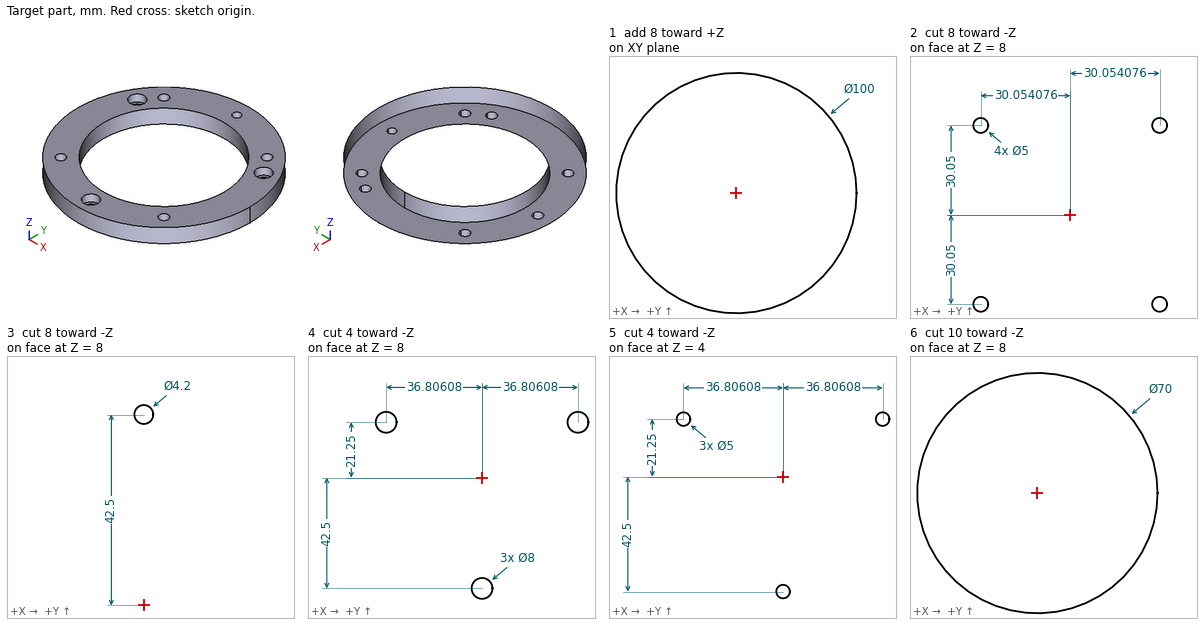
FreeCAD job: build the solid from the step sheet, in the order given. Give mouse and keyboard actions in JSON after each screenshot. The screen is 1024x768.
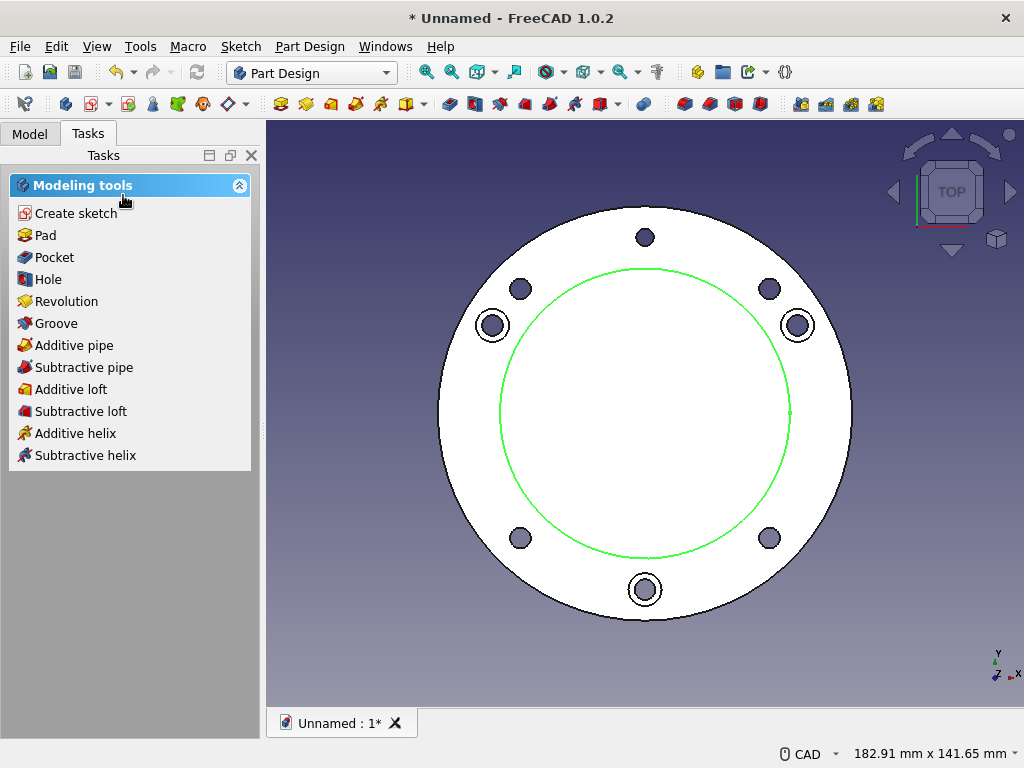
{"action": "left_click", "coordinate": [450, 104]}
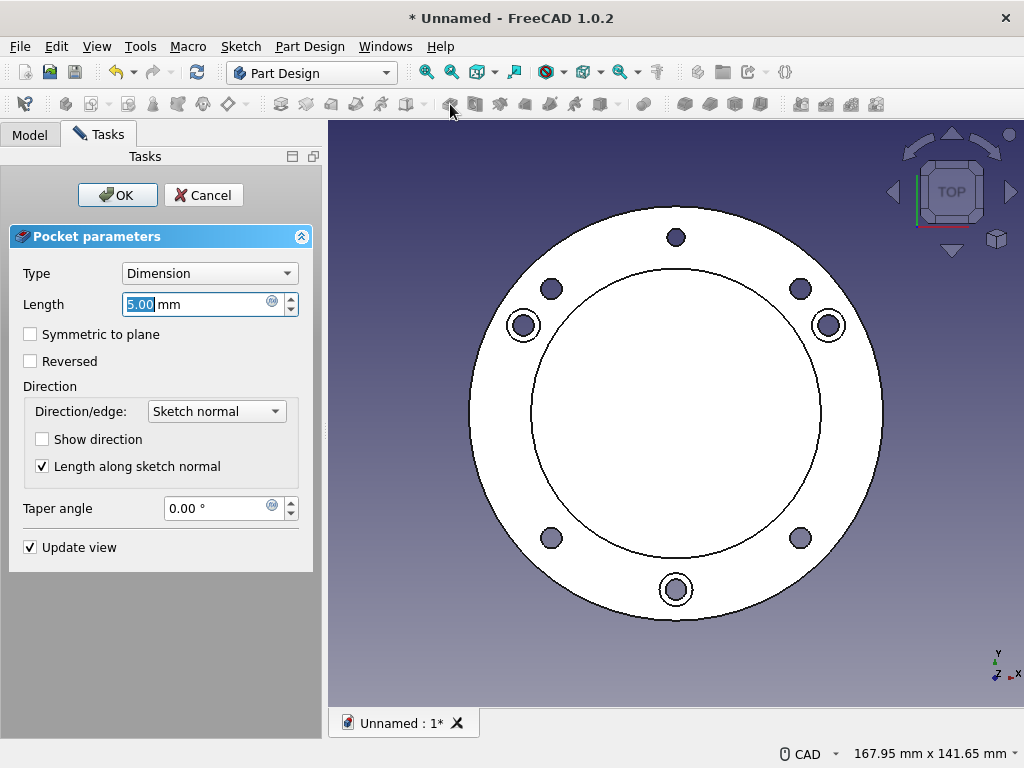
{"action": "type", "text": "10"}
{"action": "key", "text": "Tab"}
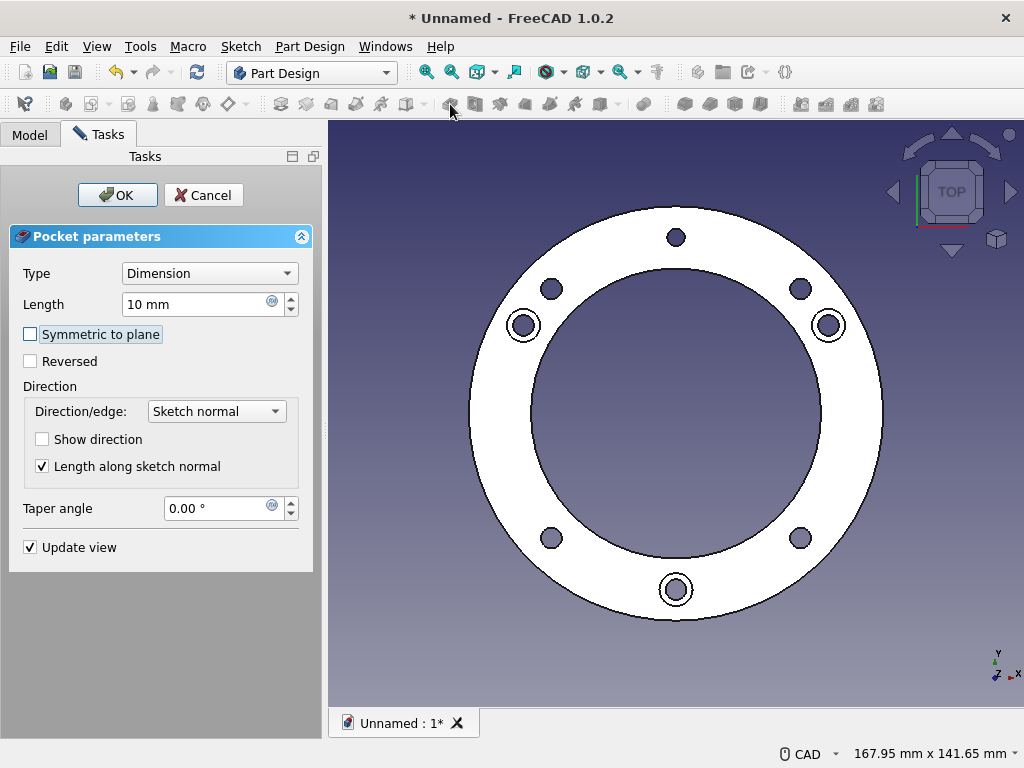
{"action": "left_click", "coordinate": [118, 195]}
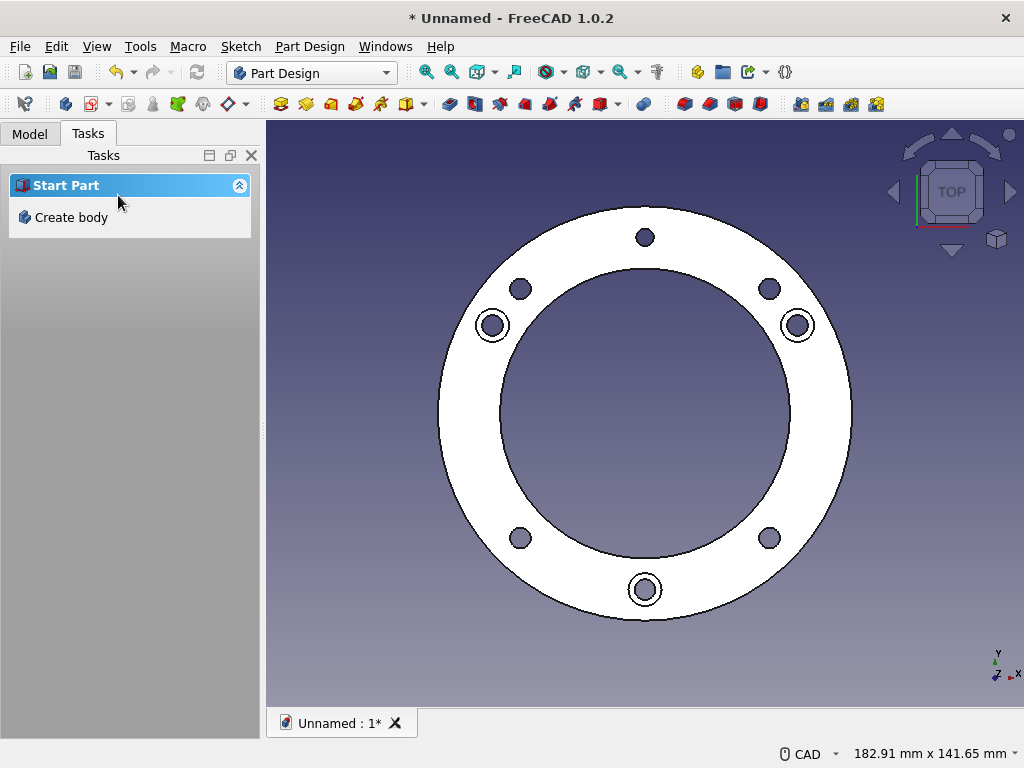
{"action": "key", "text": "0"}